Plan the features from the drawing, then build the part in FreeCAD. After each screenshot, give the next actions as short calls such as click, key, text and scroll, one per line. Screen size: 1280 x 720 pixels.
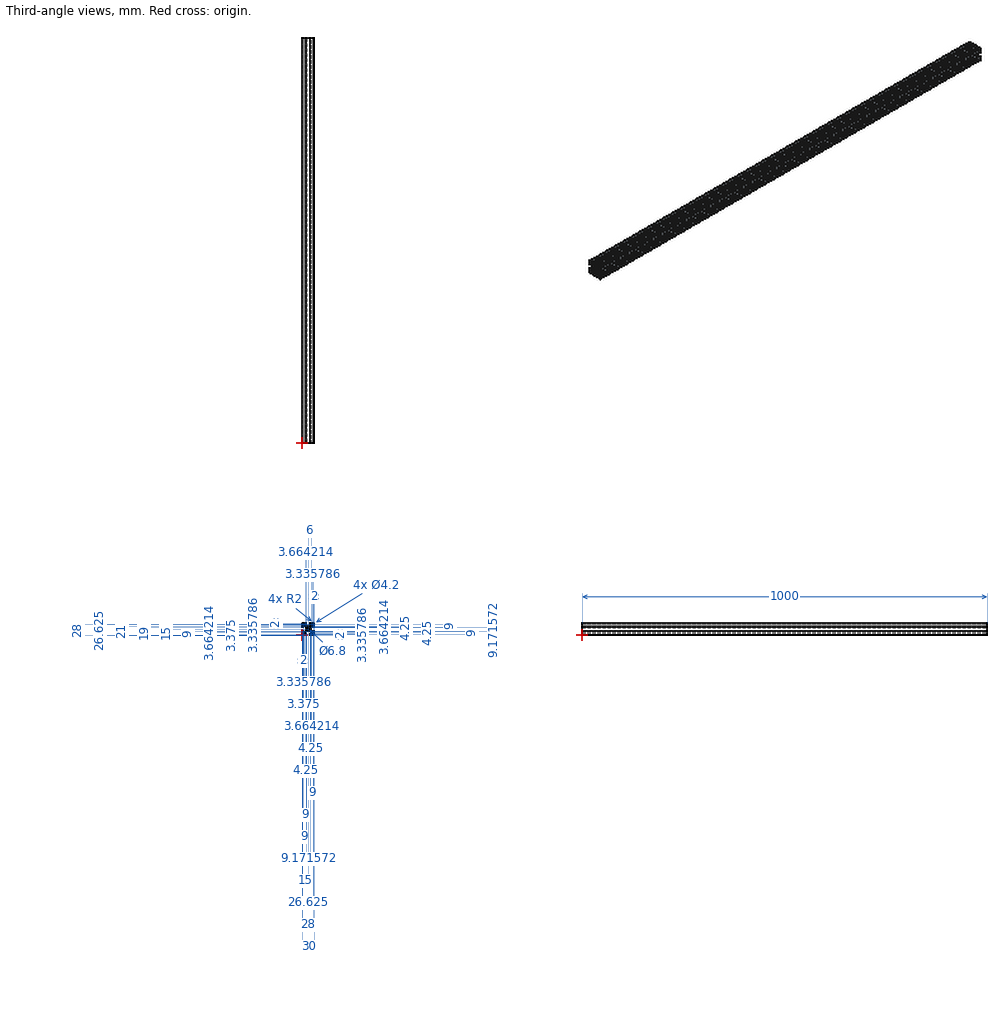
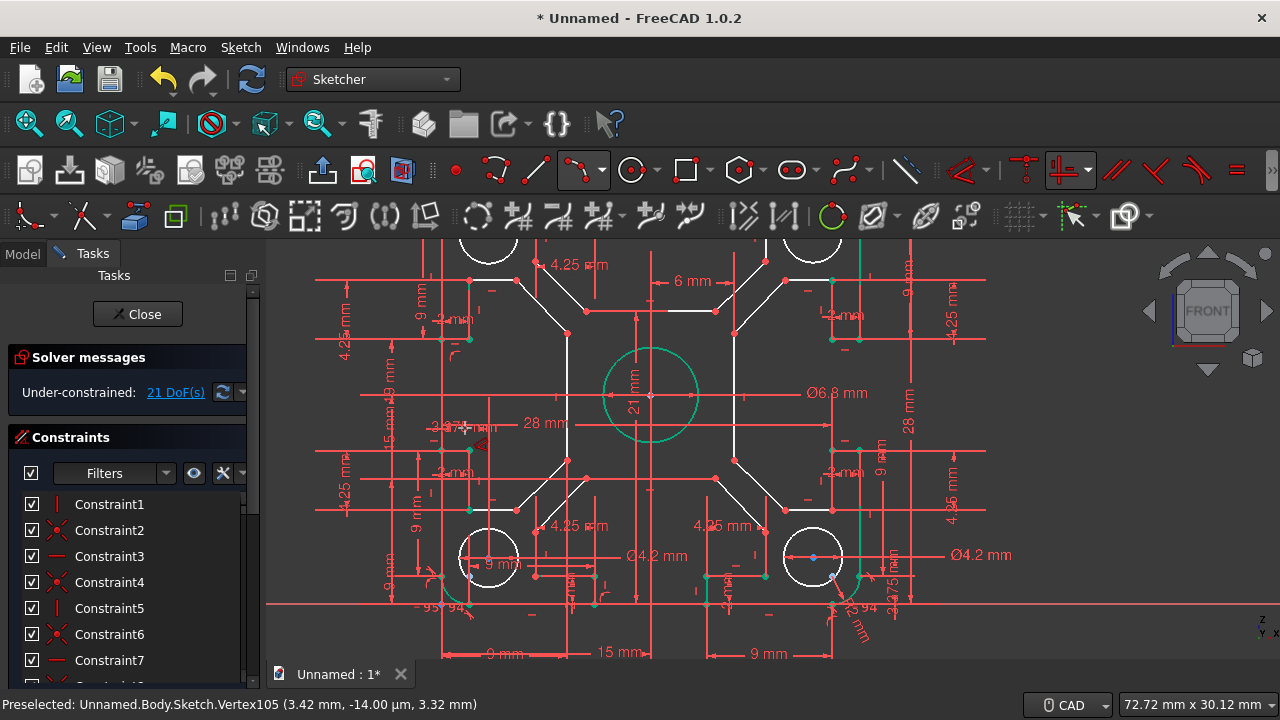
click(489, 558)
click(312, 581)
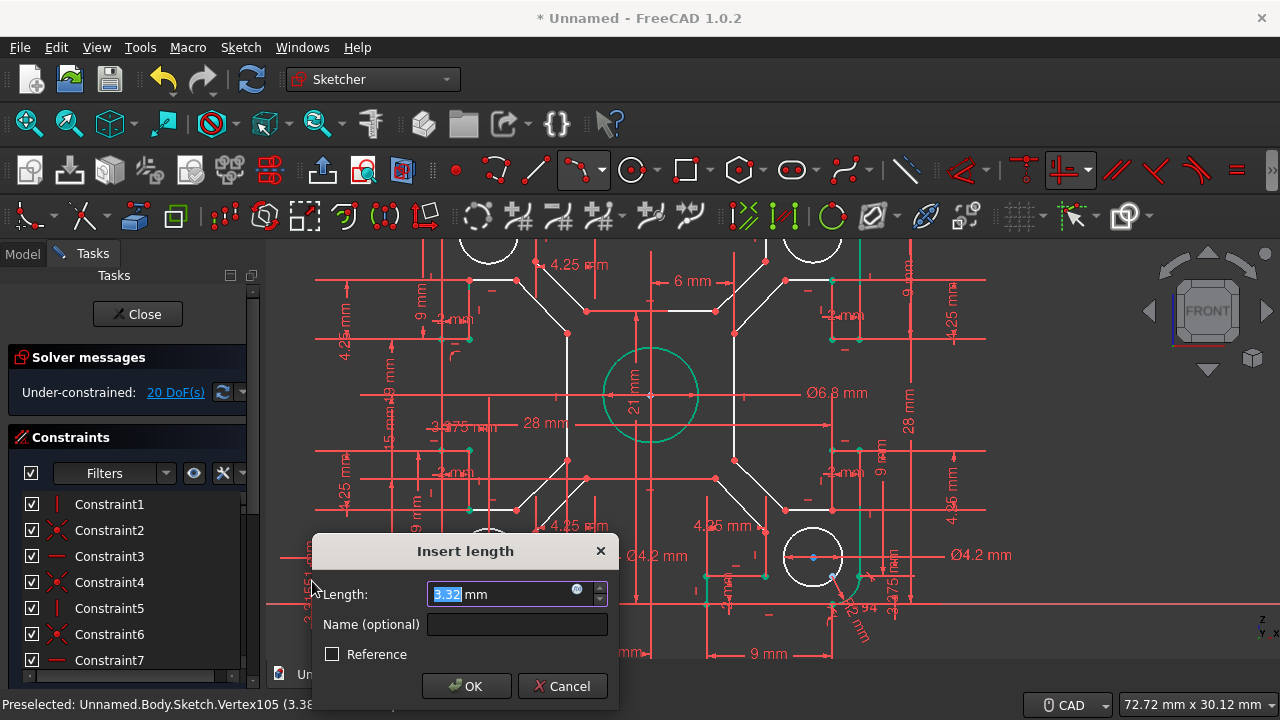
text(3.375)
key(Return)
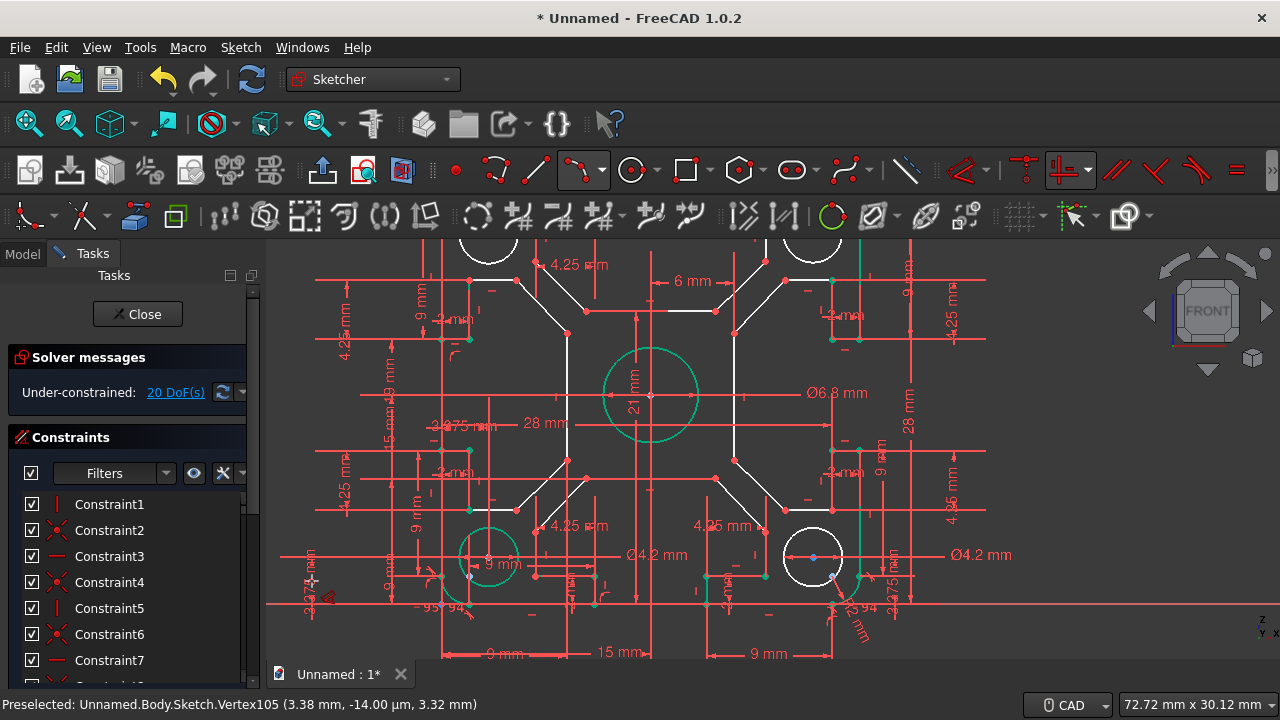
scroll(814, 559, down, 2)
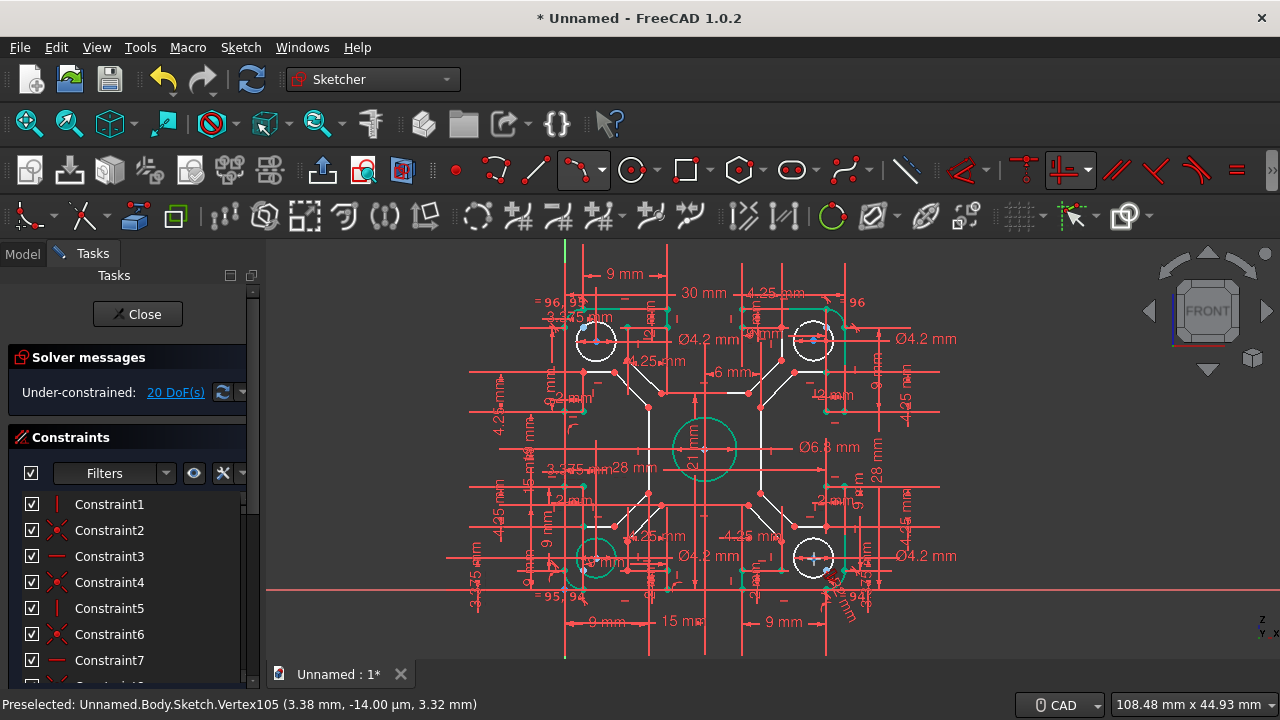
click(813, 341)
click(746, 624)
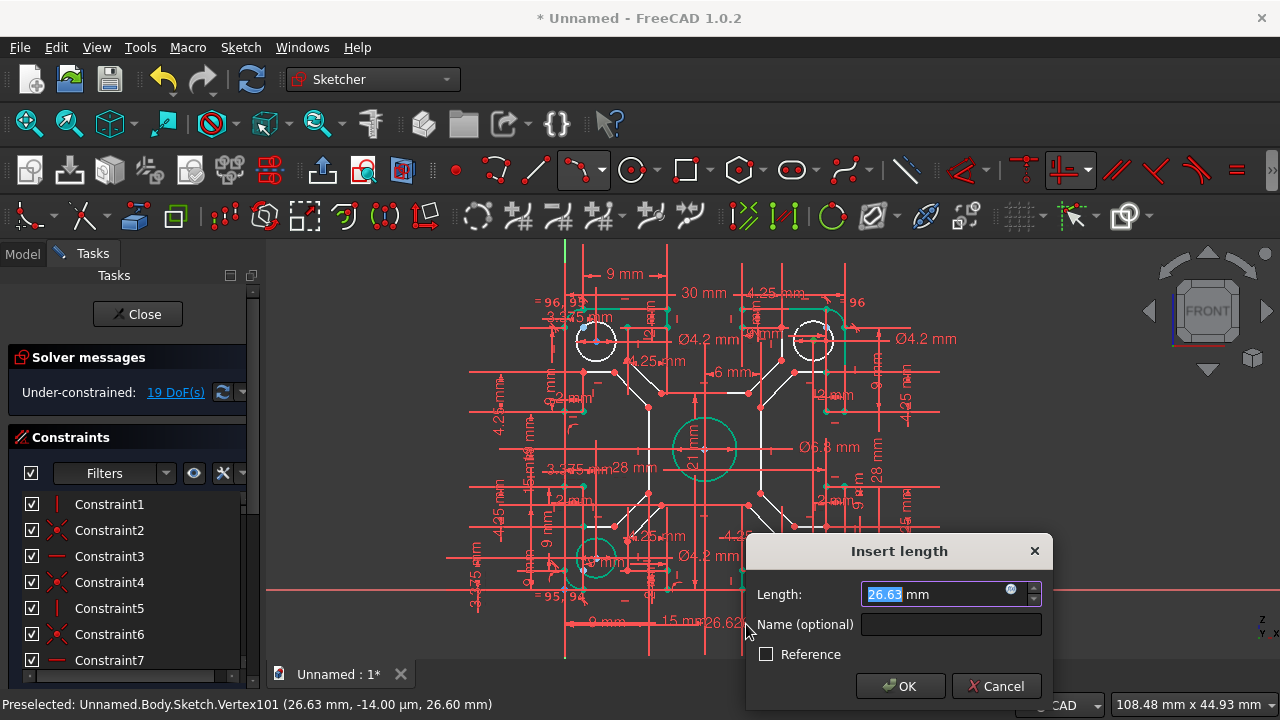
text(26.625)
key(Return)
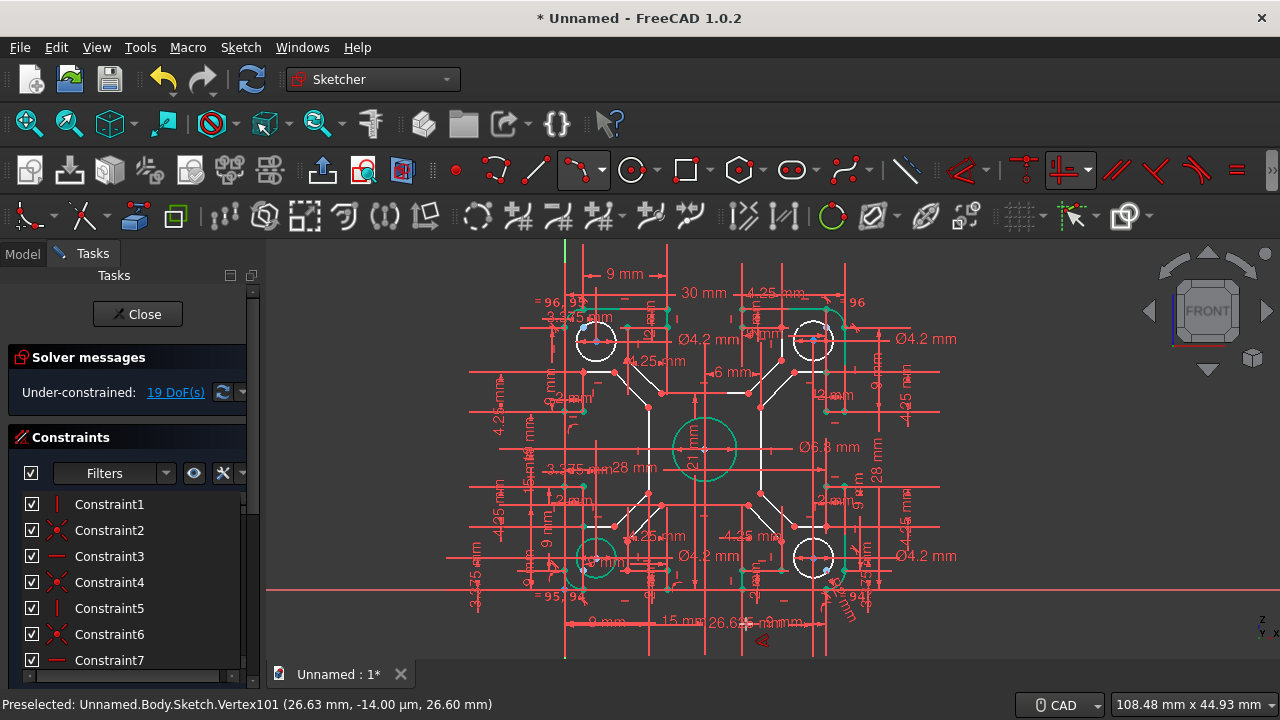
click(813, 341)
click(871, 552)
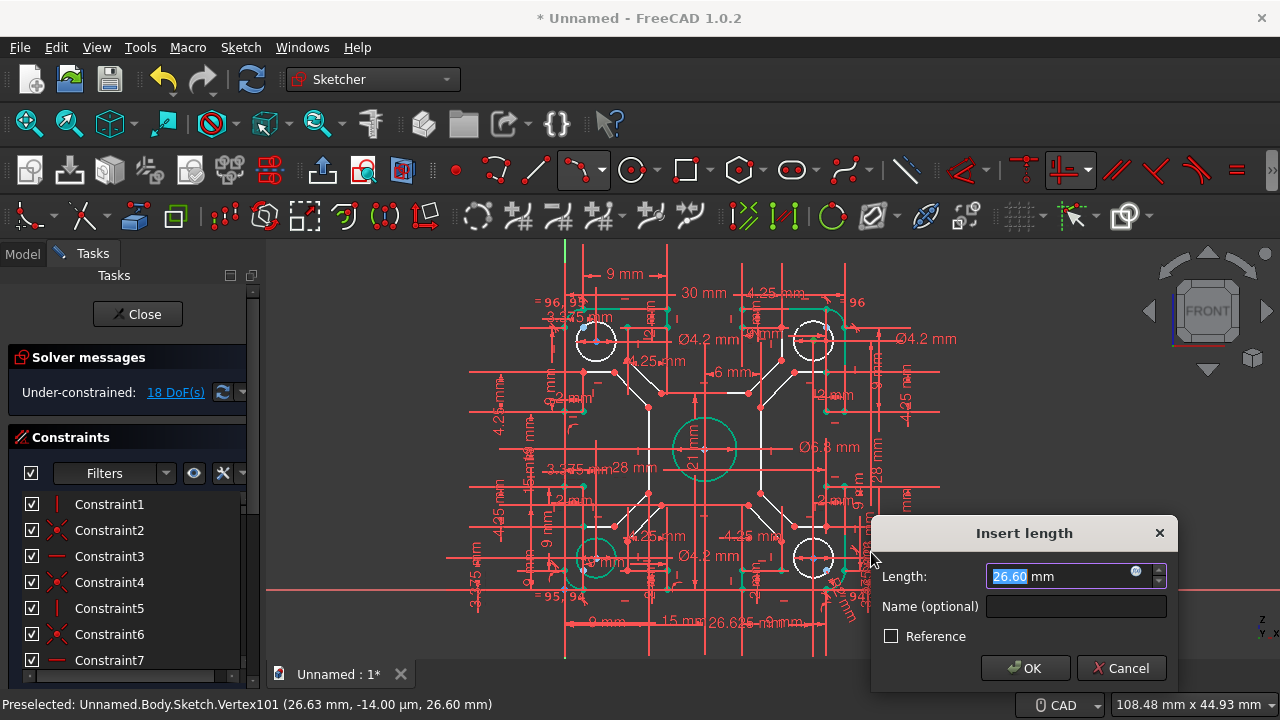
text(26.625)
key(Return)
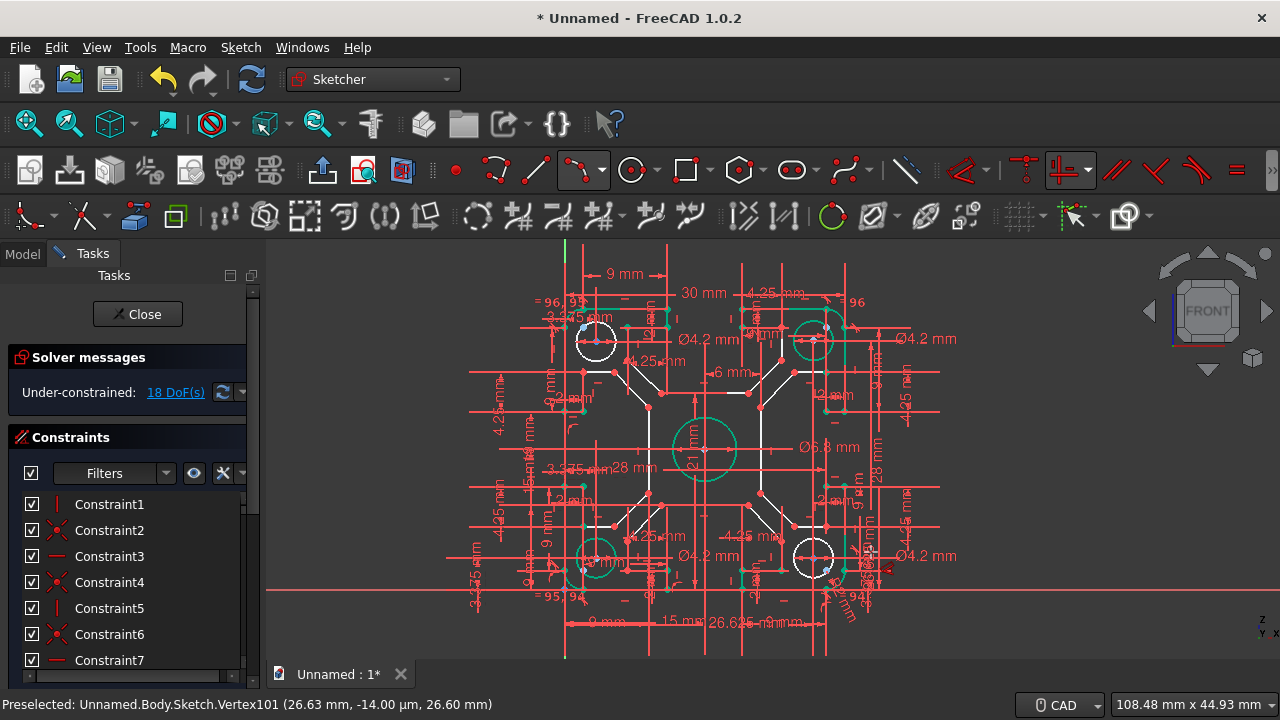
click(596, 342)
click(678, 409)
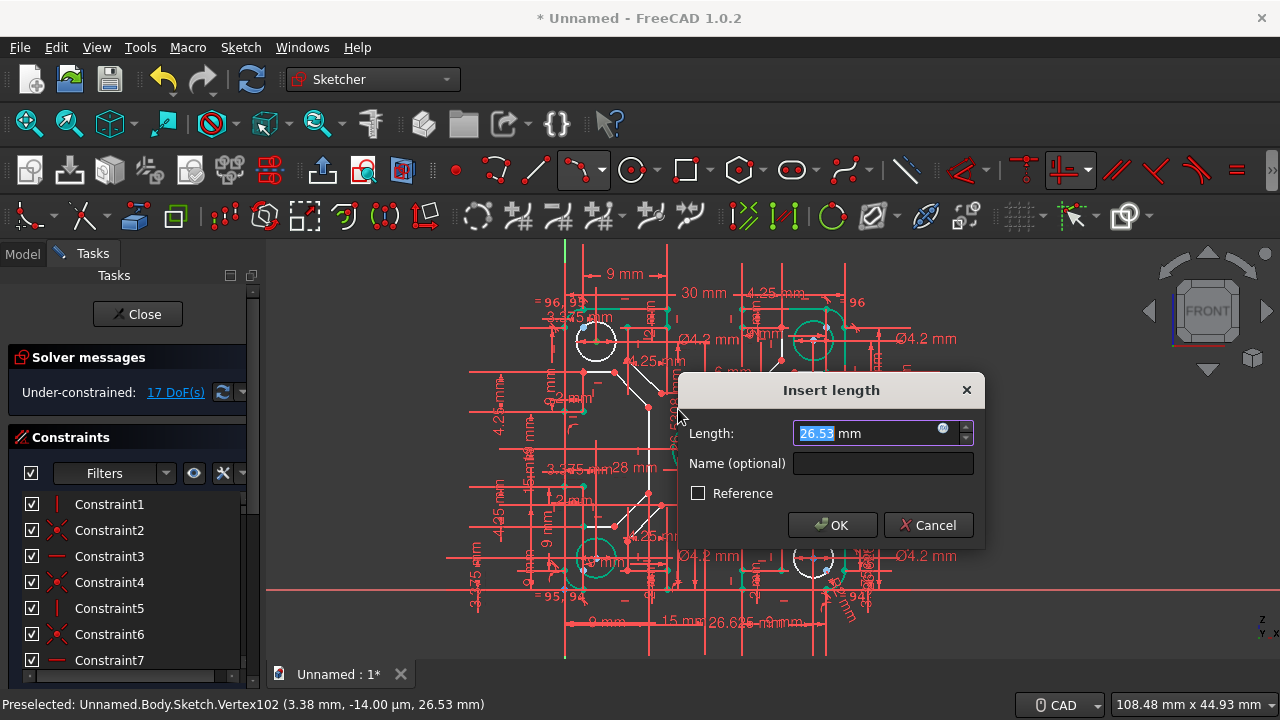
text(26.625)
key(Return)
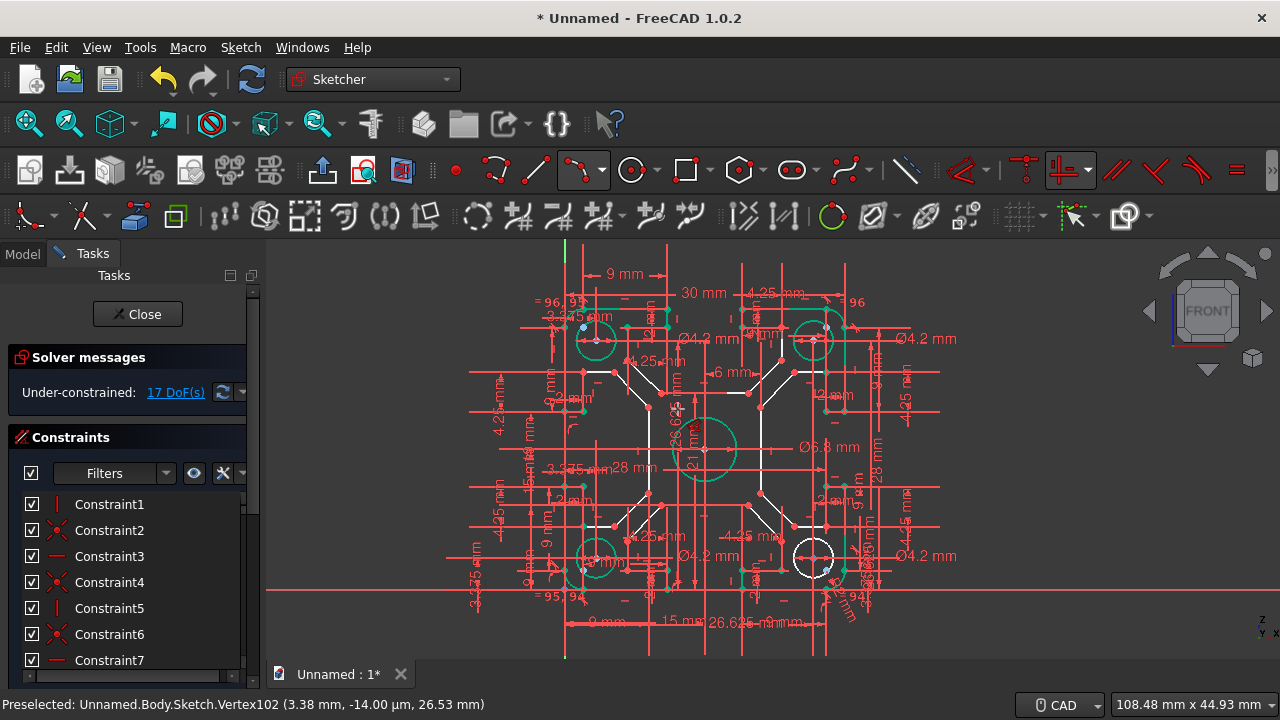
click(814, 558)
click(746, 476)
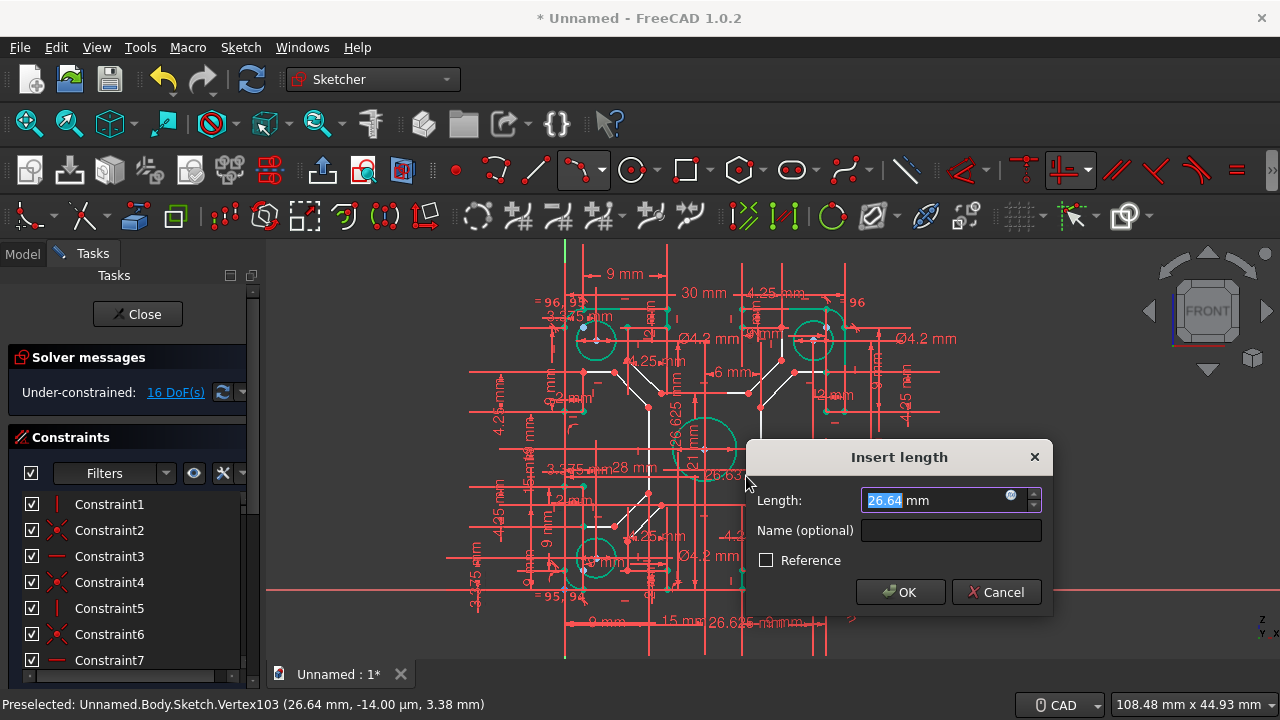
text(26.625)
key(Return)